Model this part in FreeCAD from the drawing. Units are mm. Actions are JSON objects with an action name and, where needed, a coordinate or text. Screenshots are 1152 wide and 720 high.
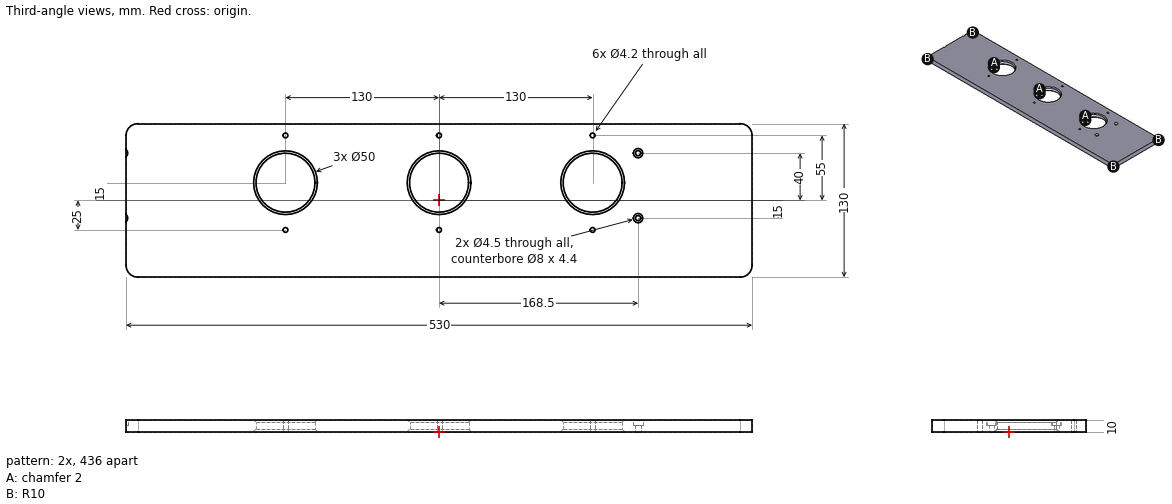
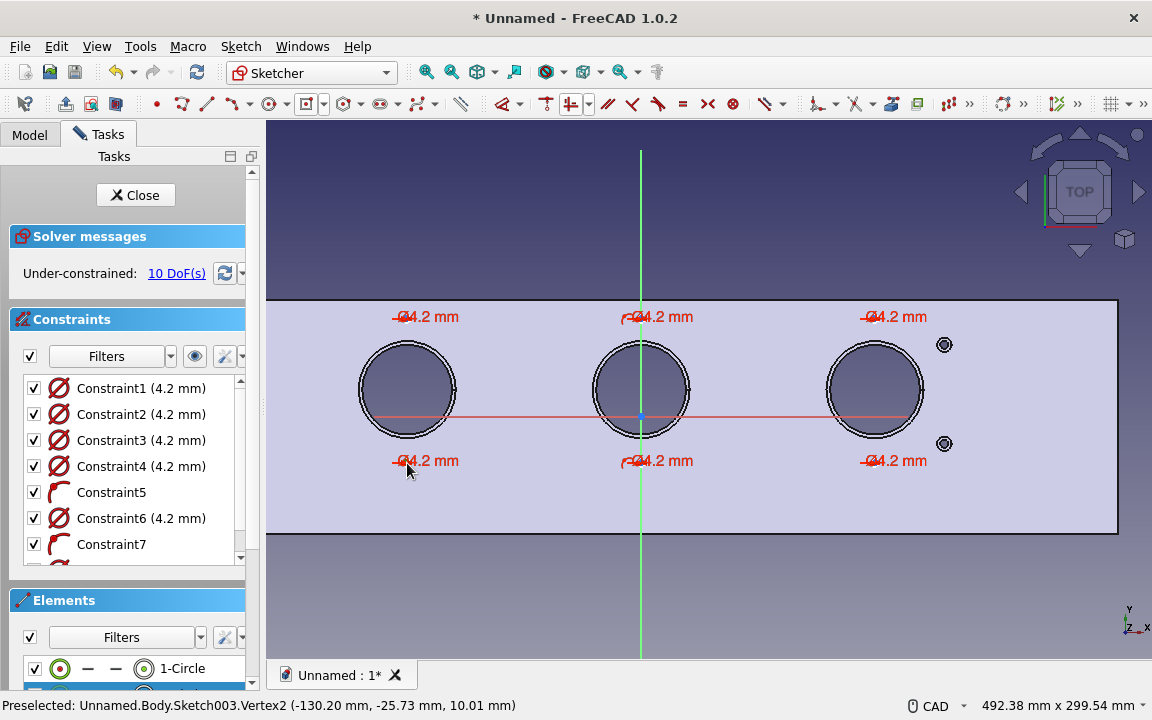
{"action": "left_click", "coordinate": [407, 319]}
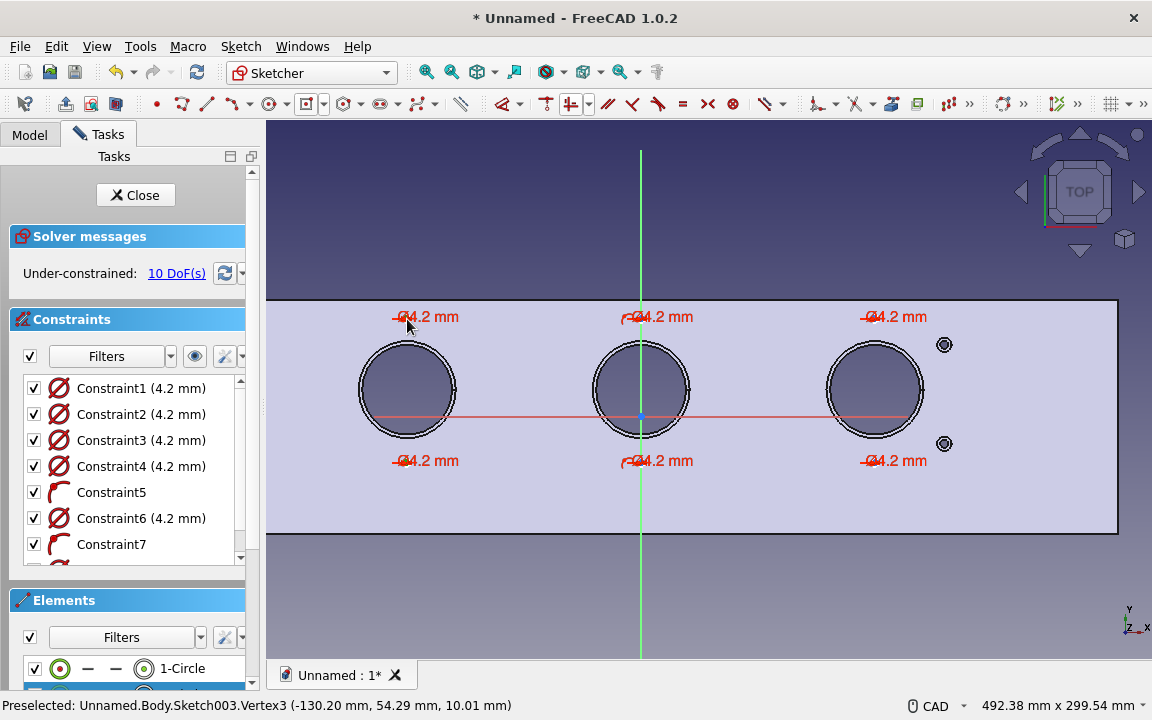
{"action": "key", "text": "v"}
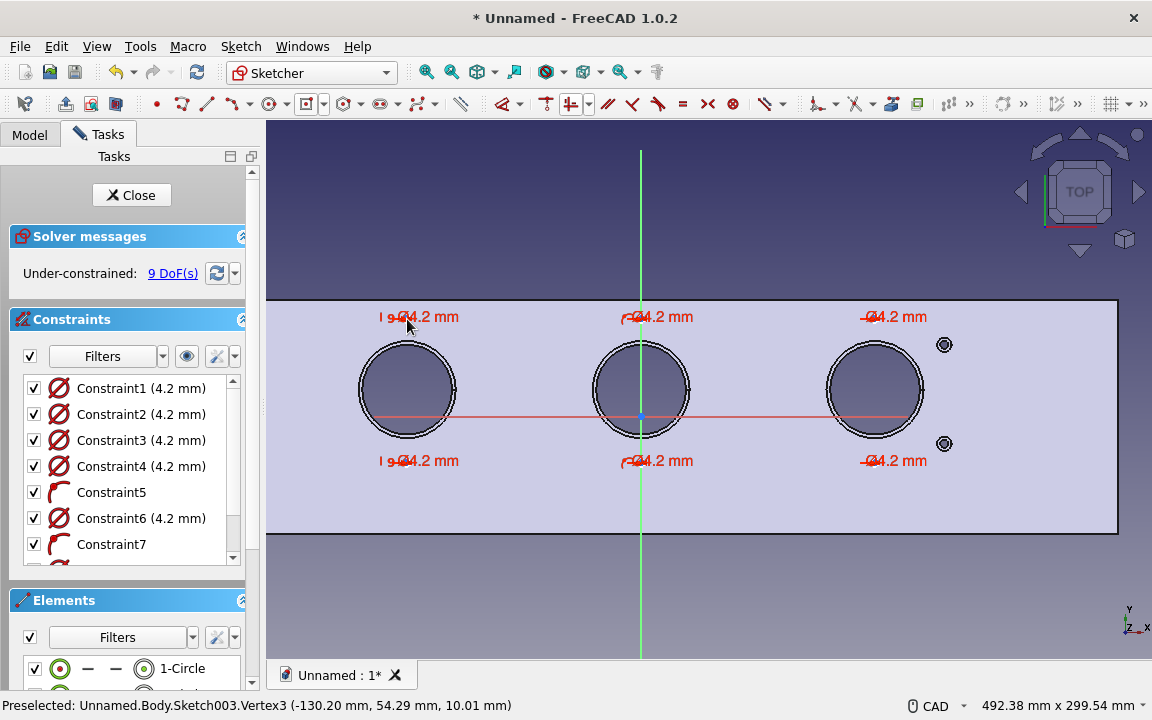
{"action": "left_click", "coordinate": [875, 319]}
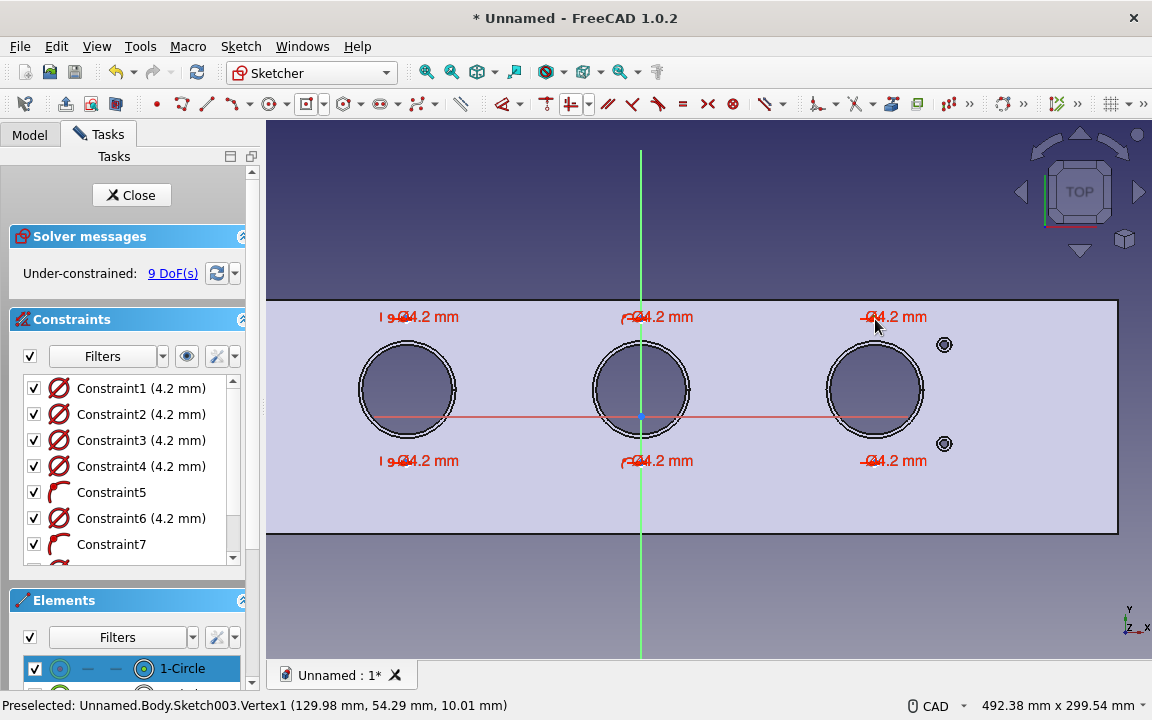
{"action": "left_click", "coordinate": [407, 319]}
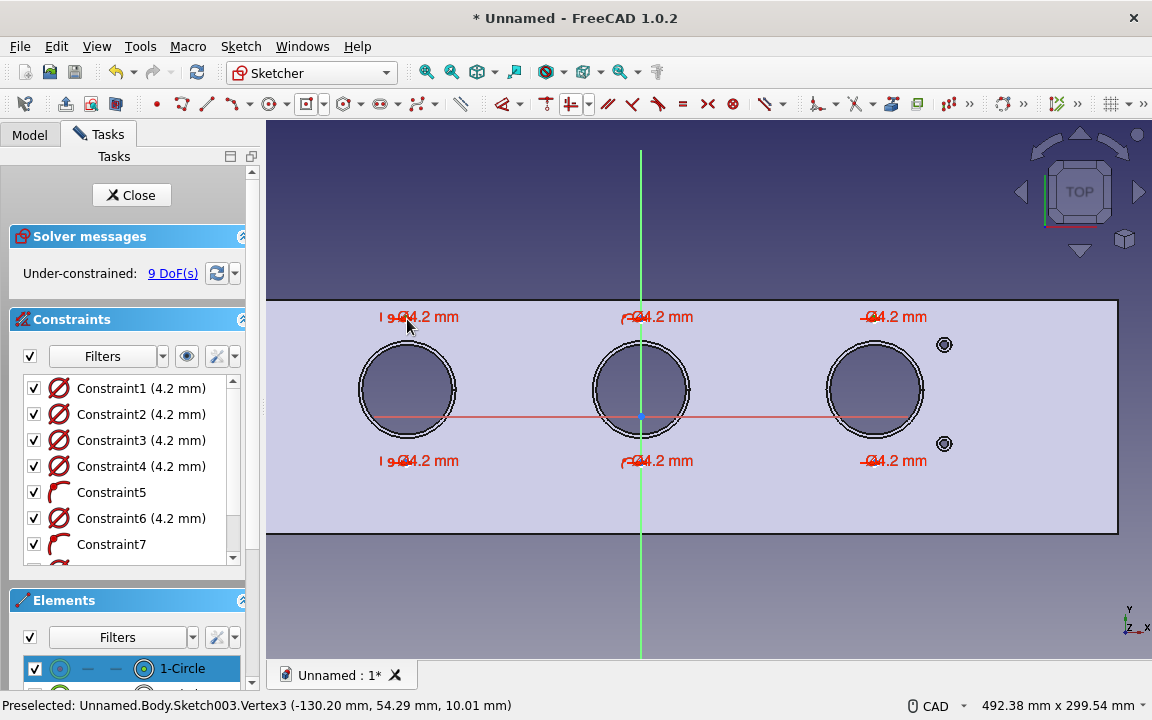
{"action": "key", "text": "h"}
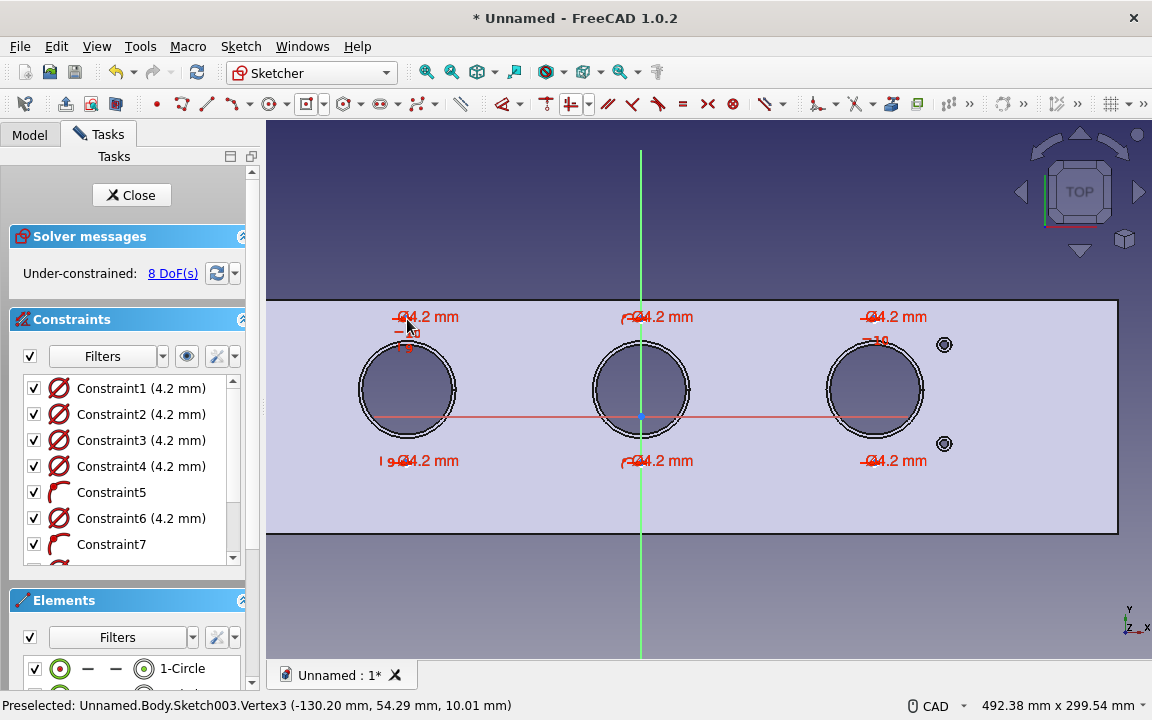
{"action": "left_click", "coordinate": [875, 319]}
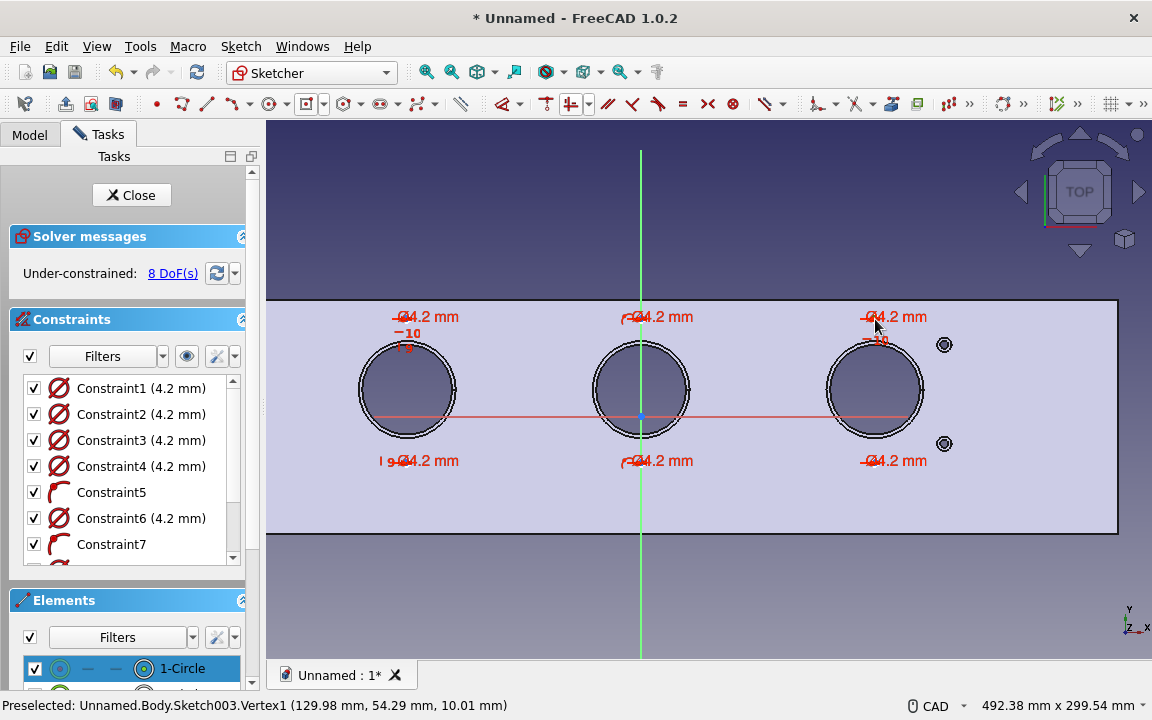
{"action": "left_click", "coordinate": [641, 319]}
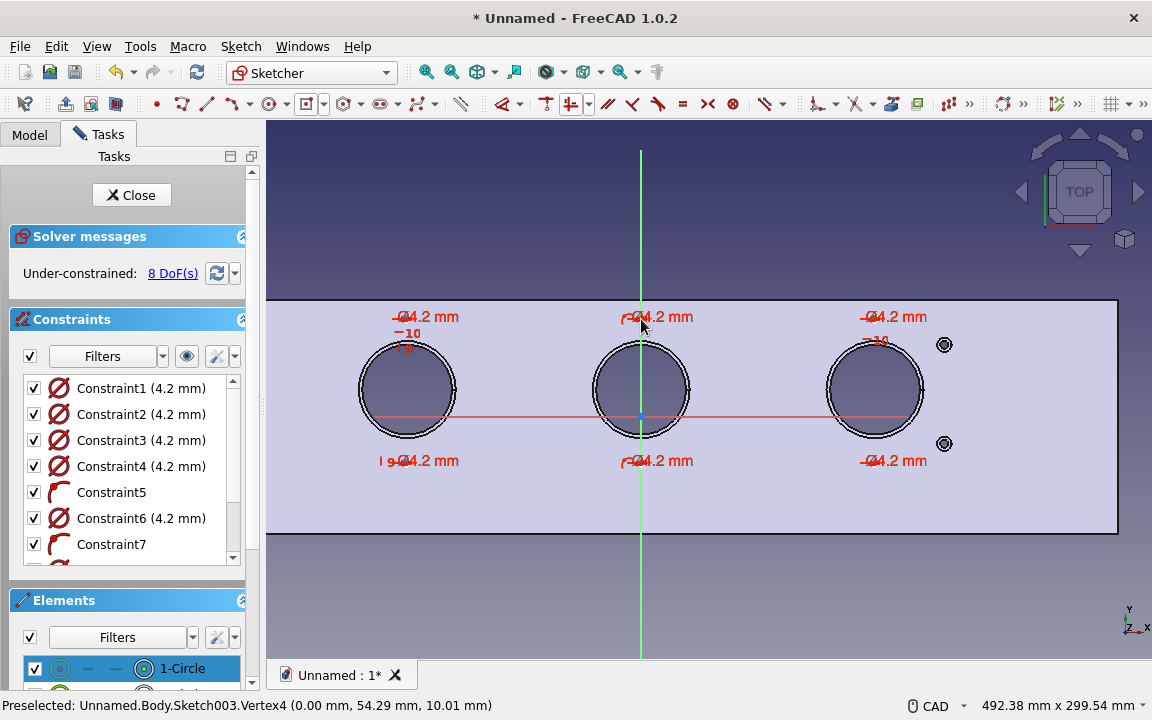
{"action": "key", "text": "h"}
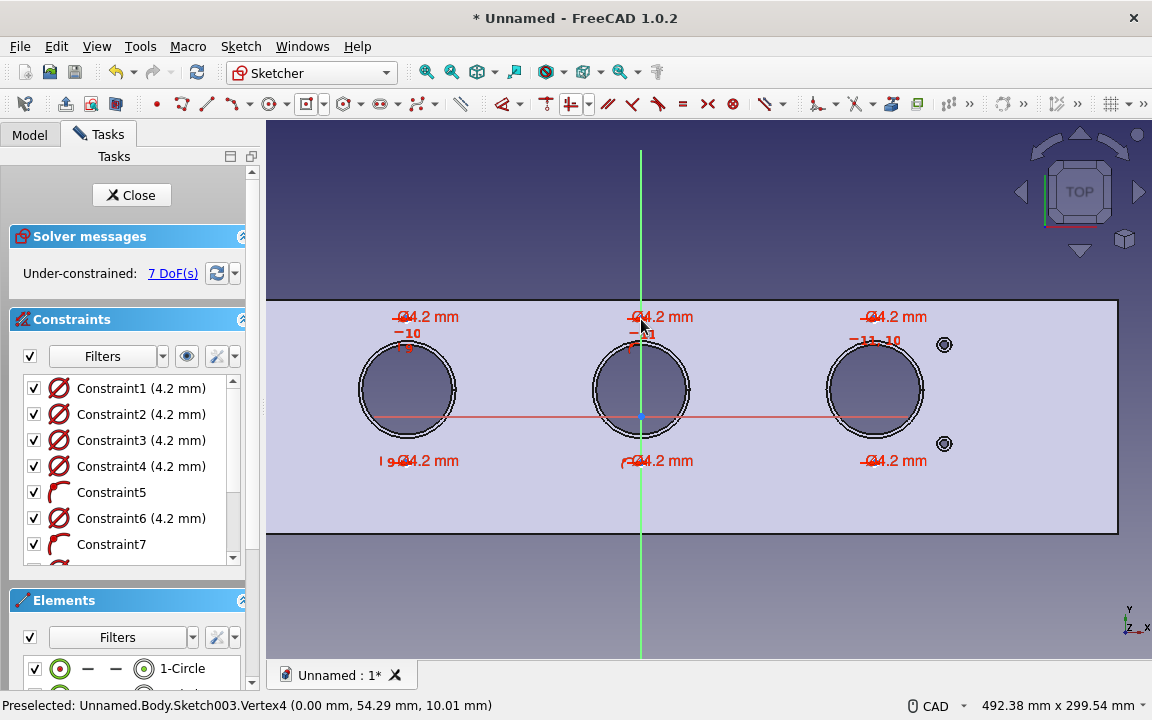
{"action": "left_click", "coordinate": [407, 463]}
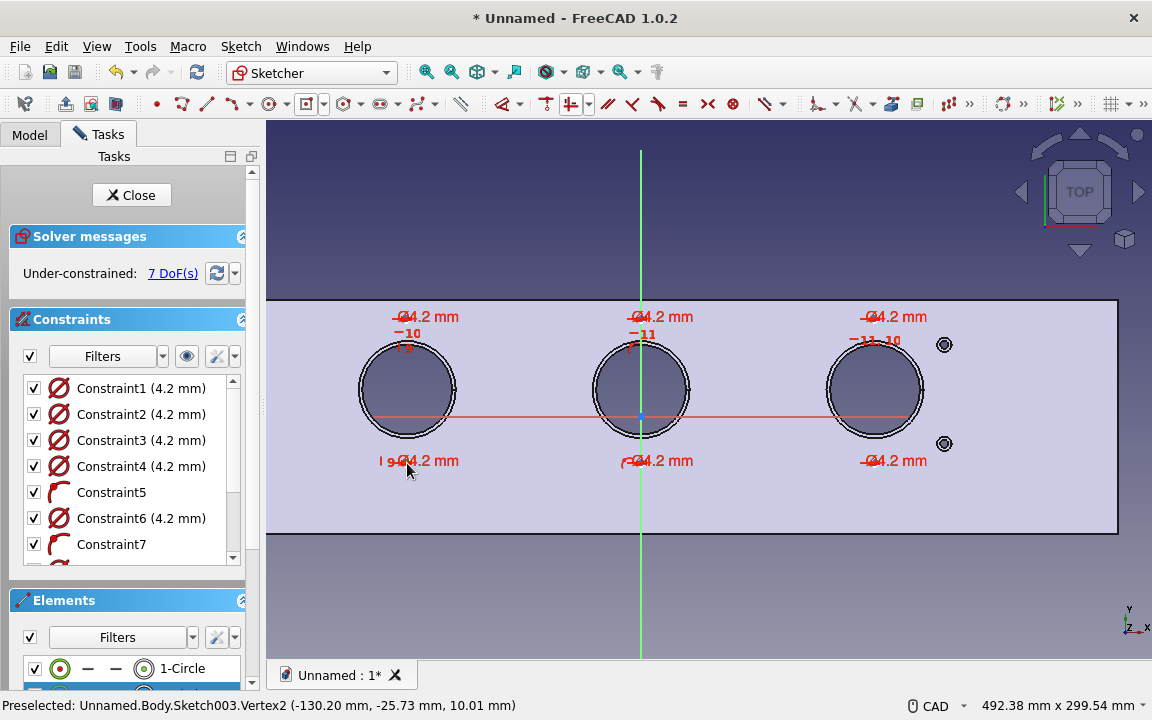
{"action": "left_click", "coordinate": [641, 463]}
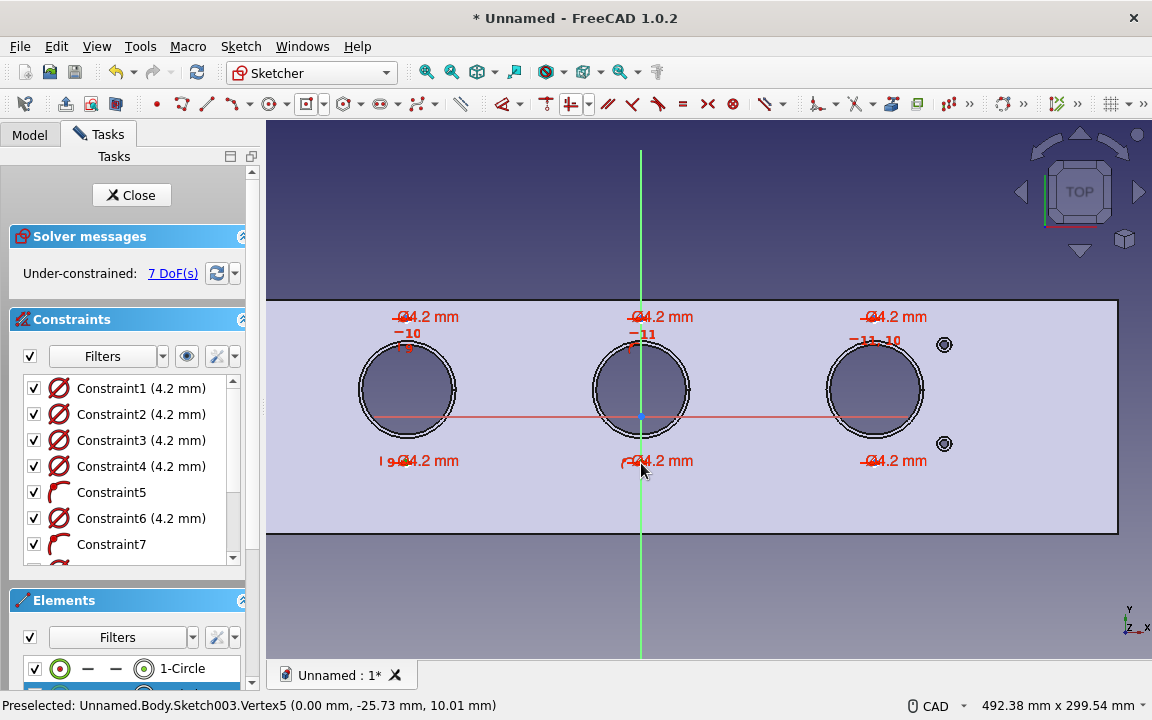
{"action": "key", "text": "h"}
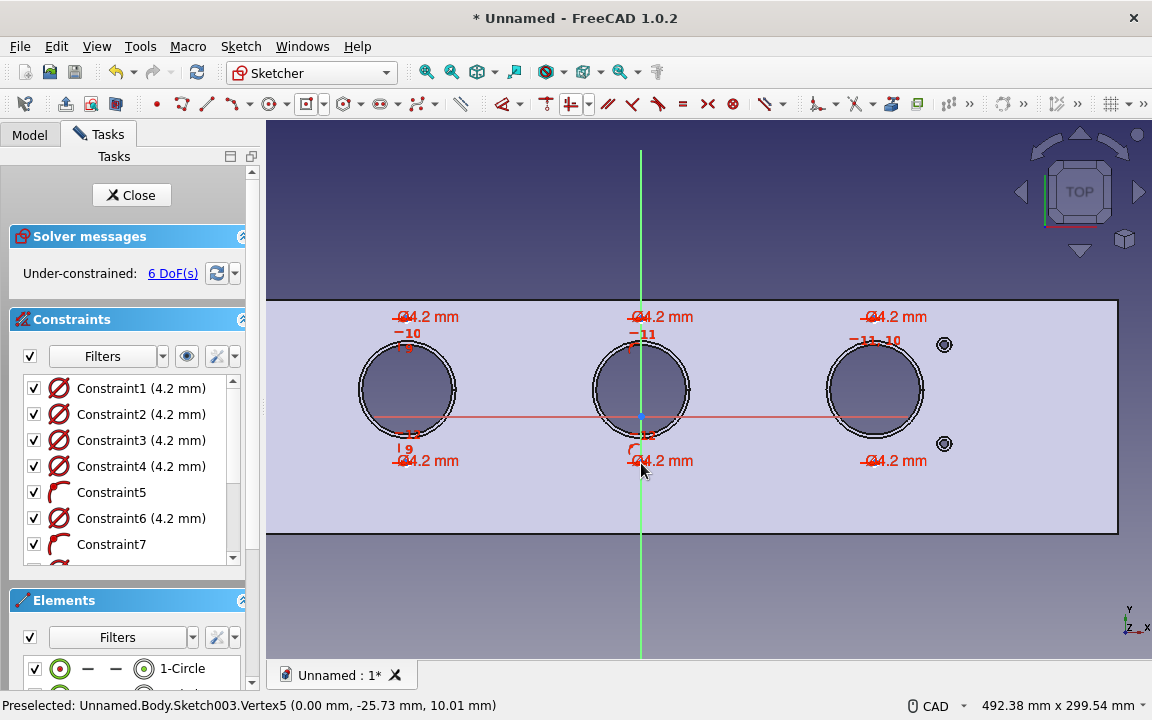
{"action": "left_click", "coordinate": [875, 319]}